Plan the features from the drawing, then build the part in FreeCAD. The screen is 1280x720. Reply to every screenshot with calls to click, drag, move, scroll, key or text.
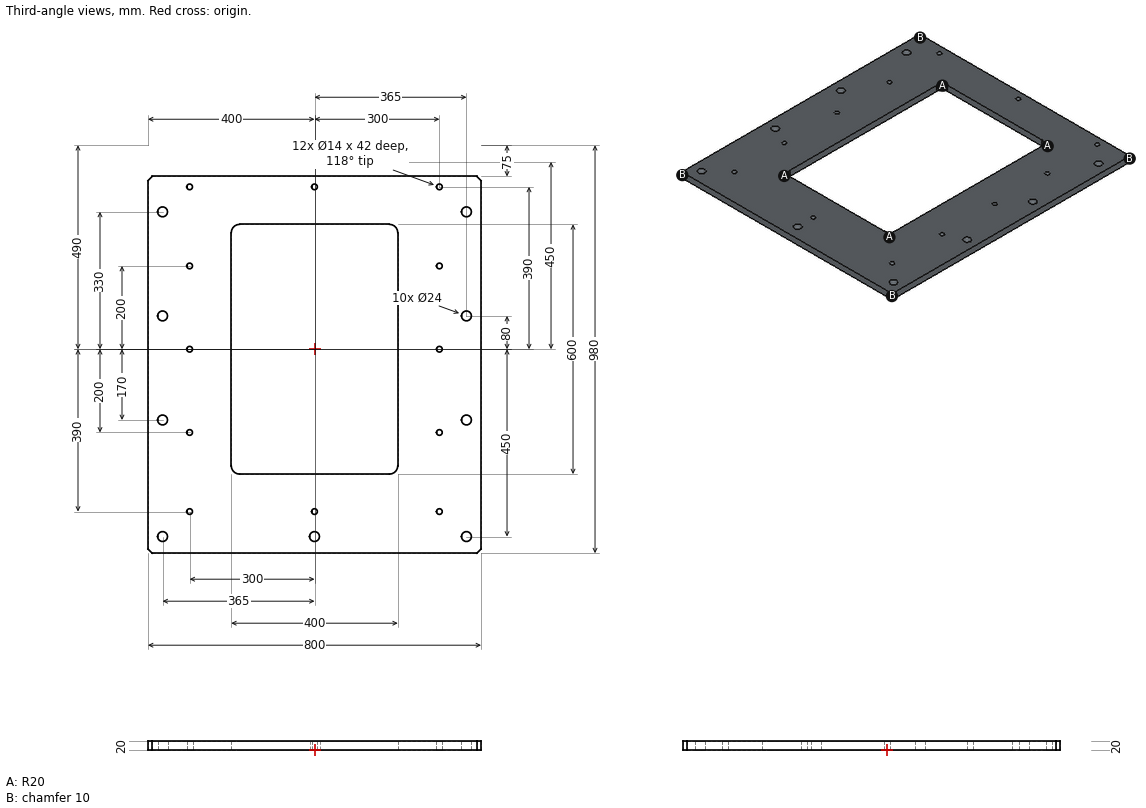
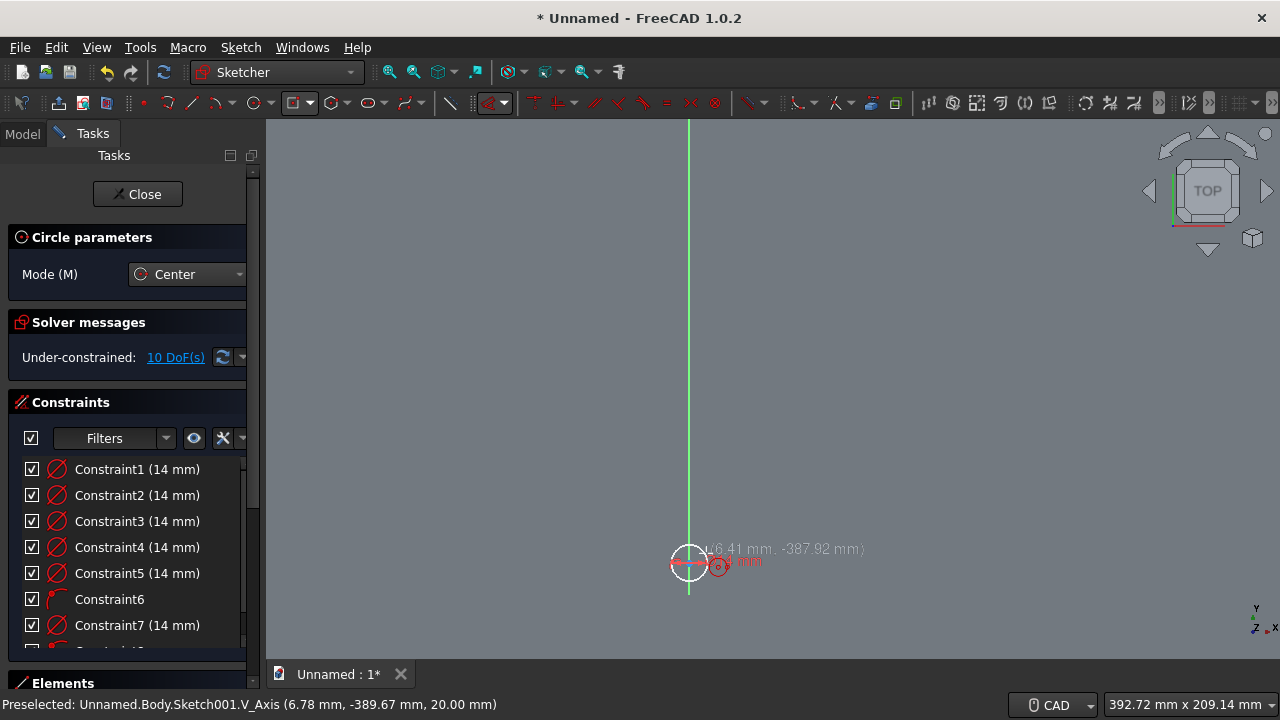
scroll(707, 555, down, 9)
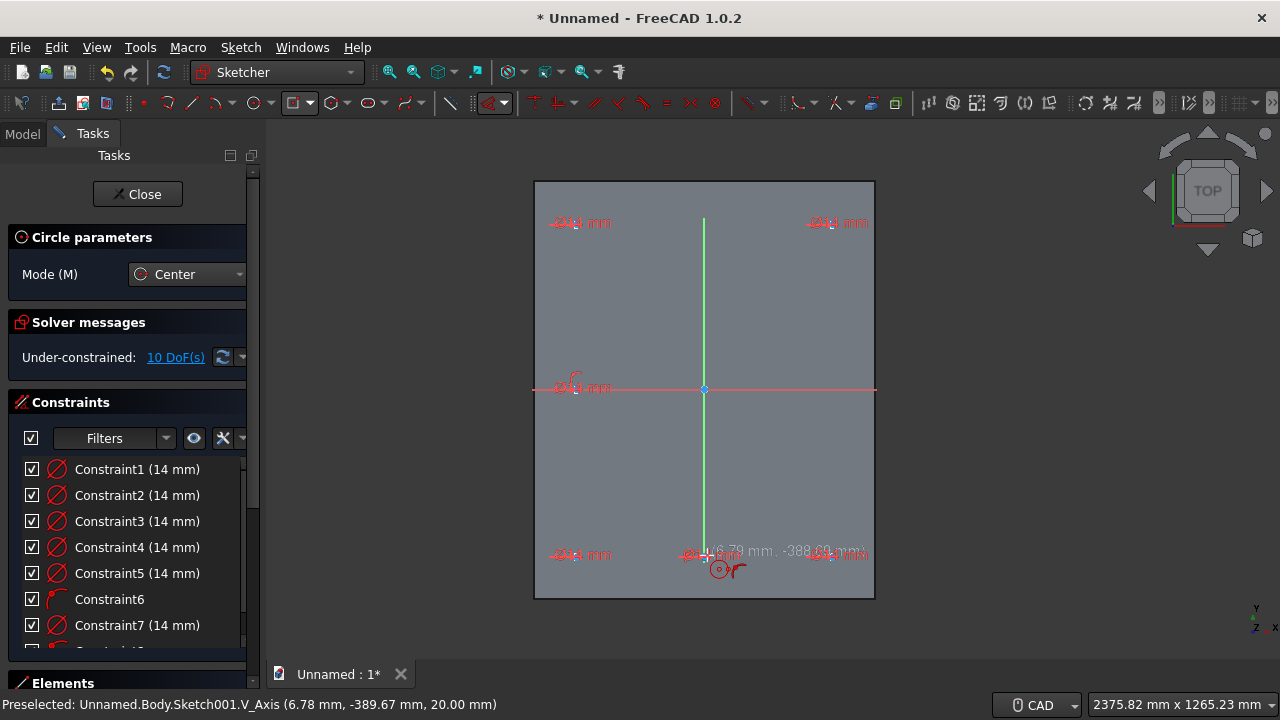
scroll(833, 390, up, 11)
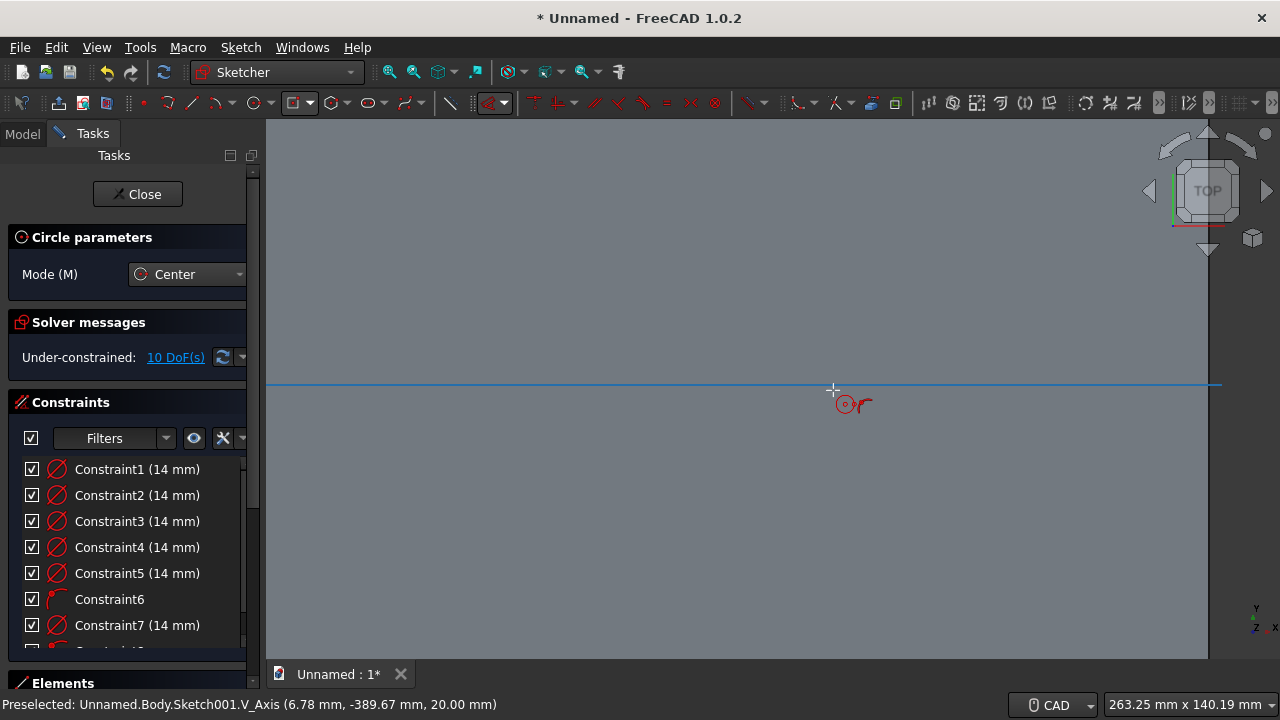
scroll(834, 389, down, 11)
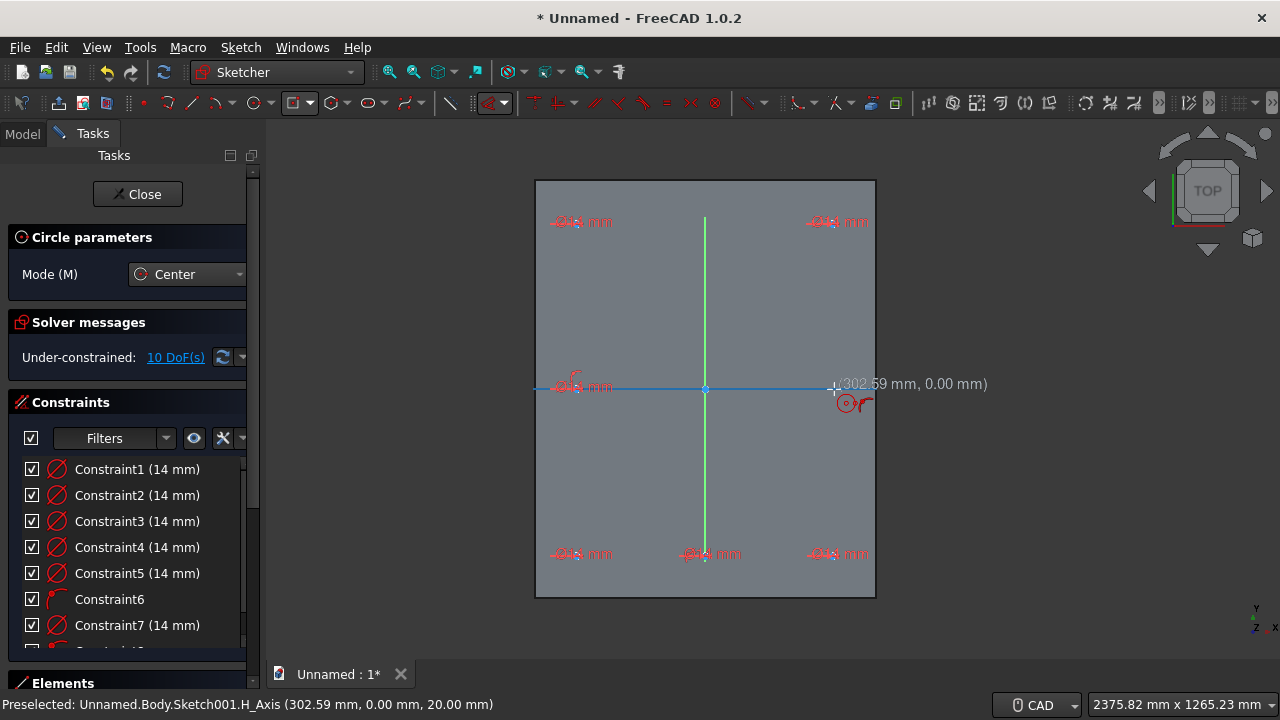
click(833, 389)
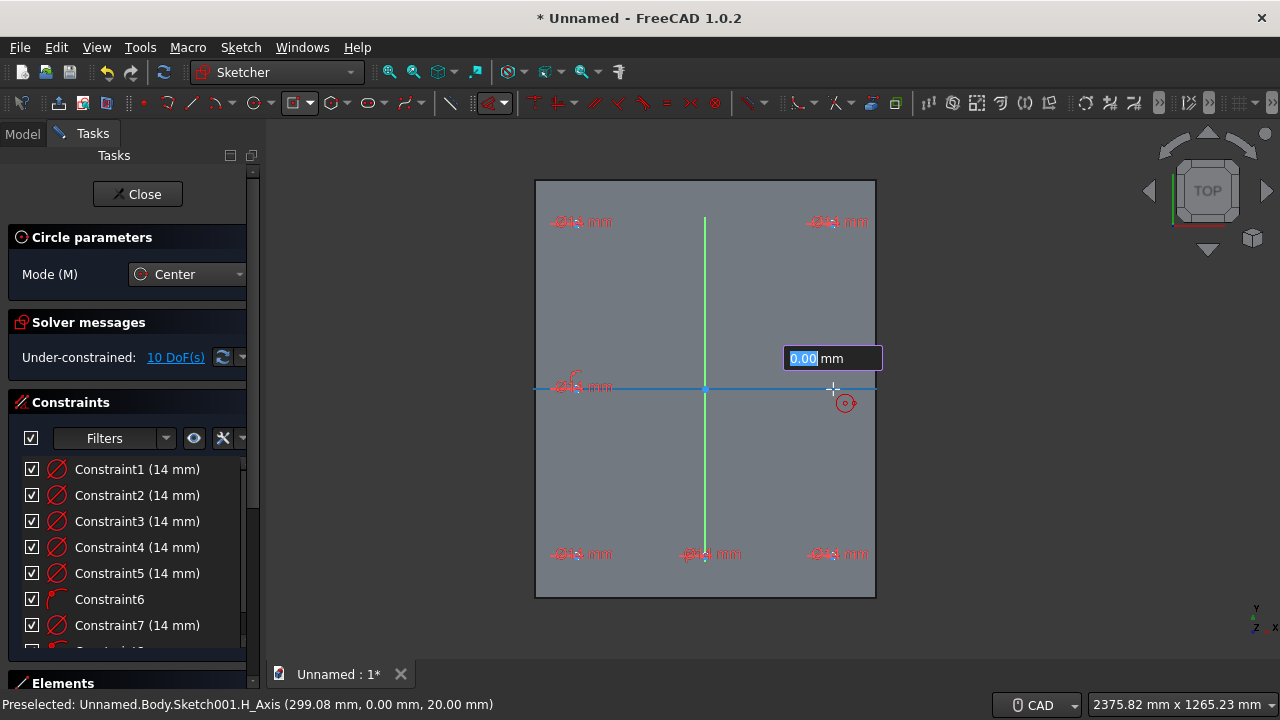
scroll(834, 386, up, 9)
move(834, 385)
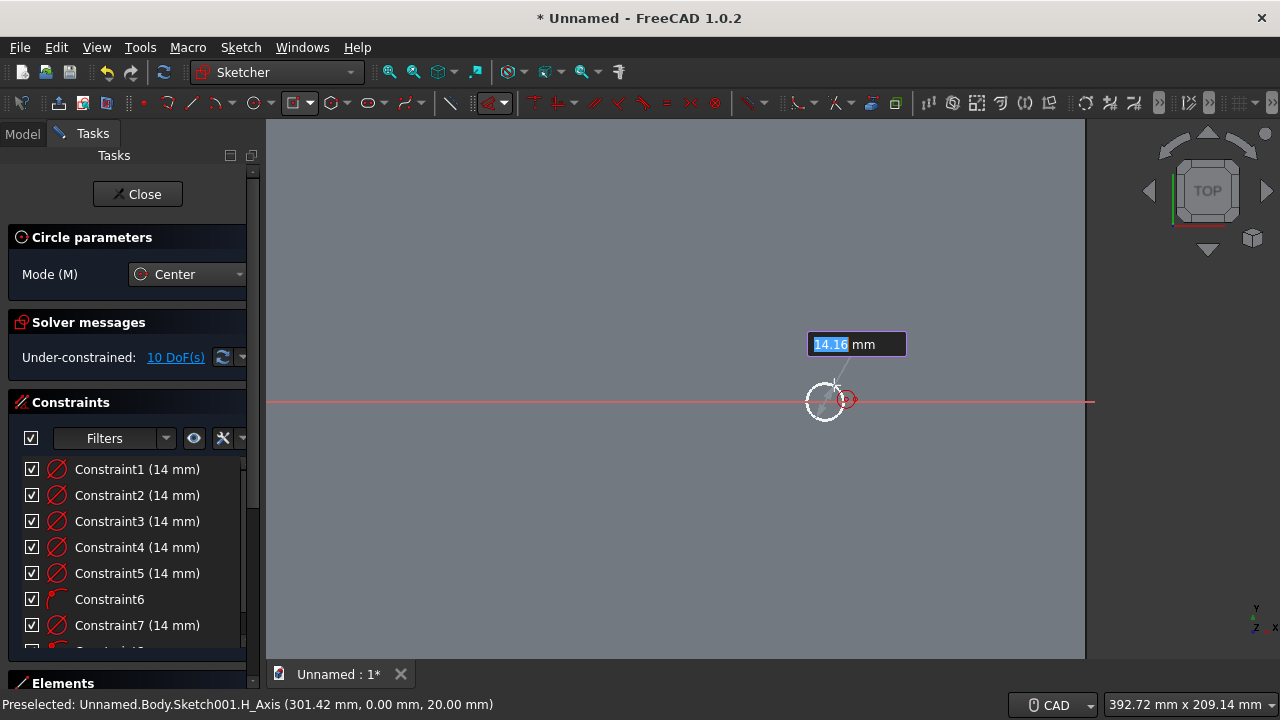
text(14)
key(Return)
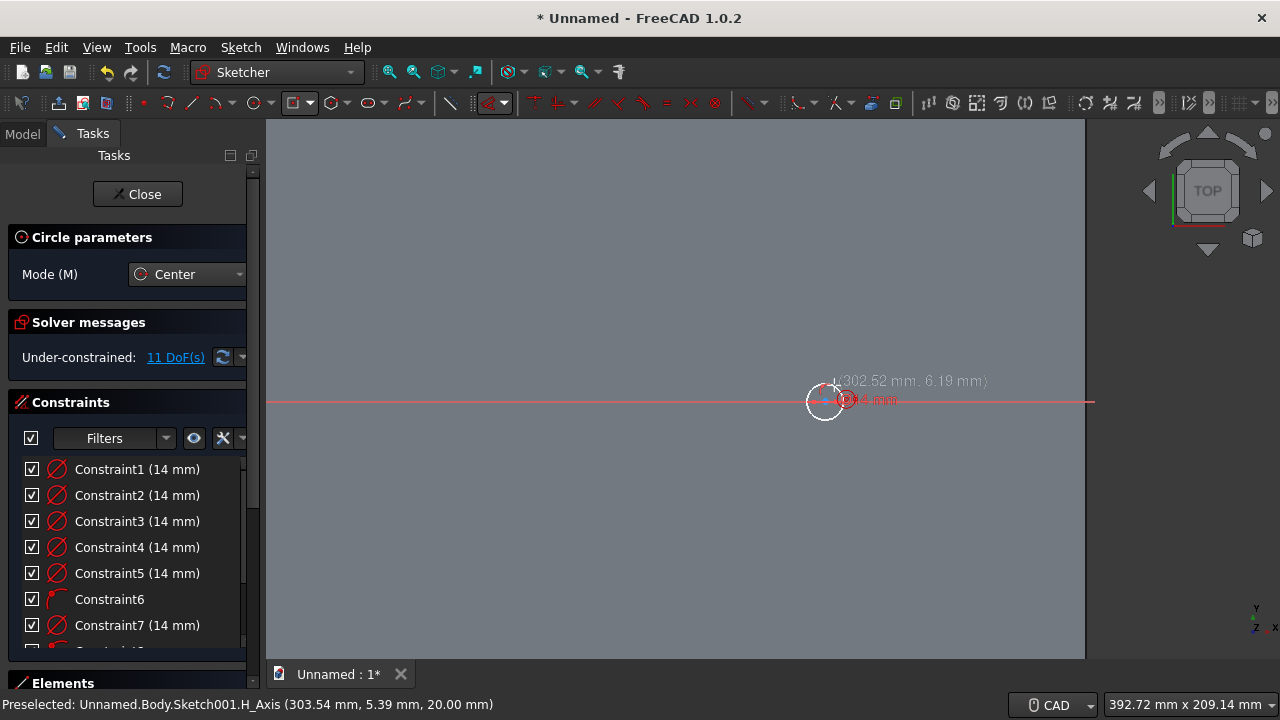
scroll(834, 386, down, 9)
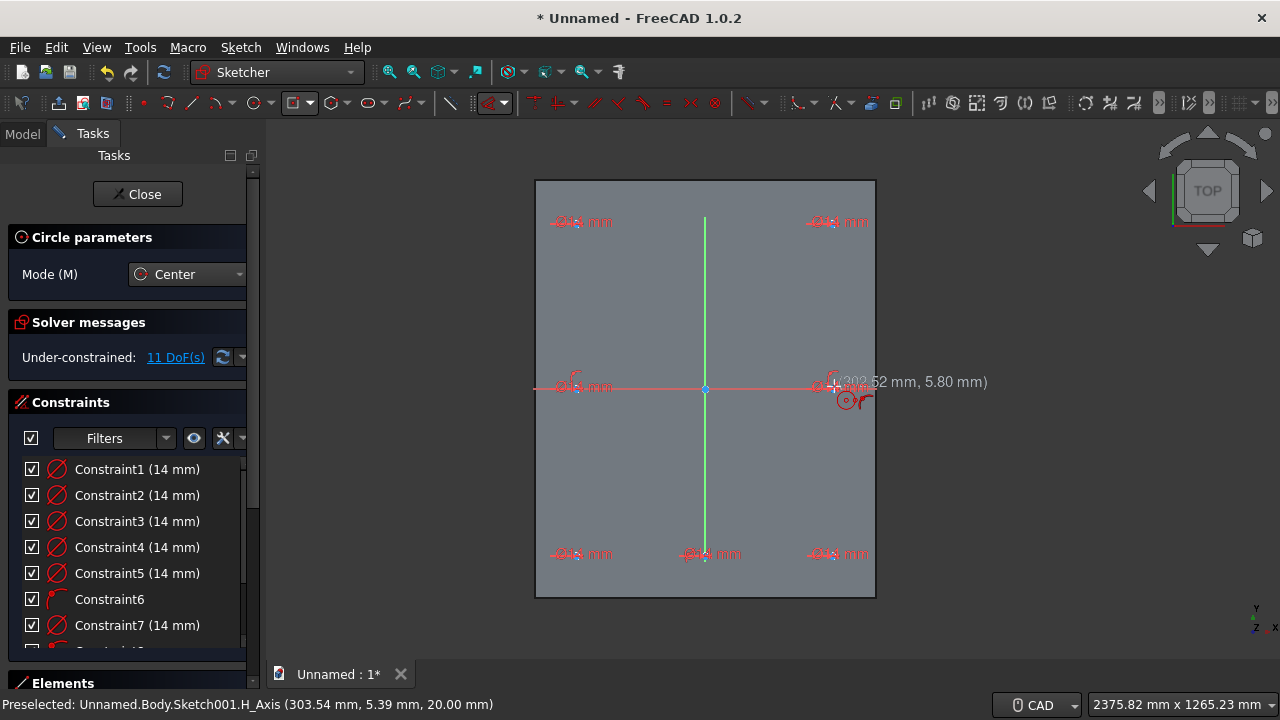
scroll(705, 223, up, 11)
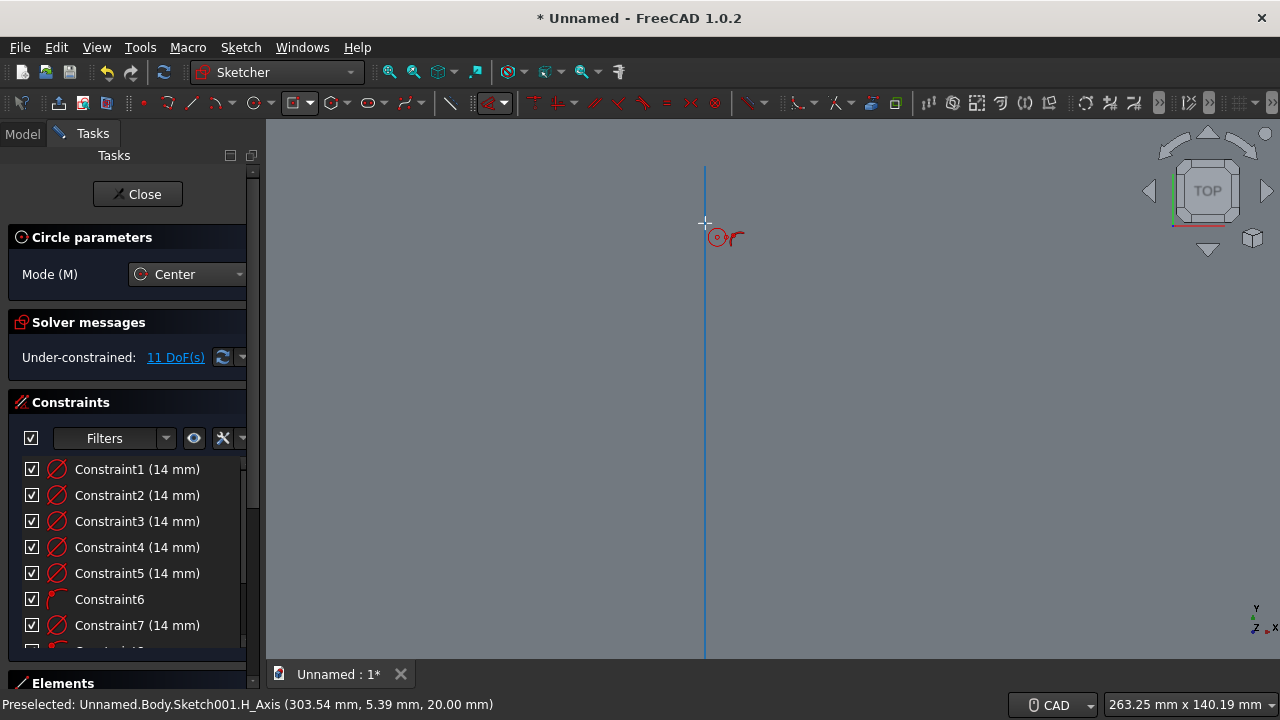
scroll(704, 223, down, 11)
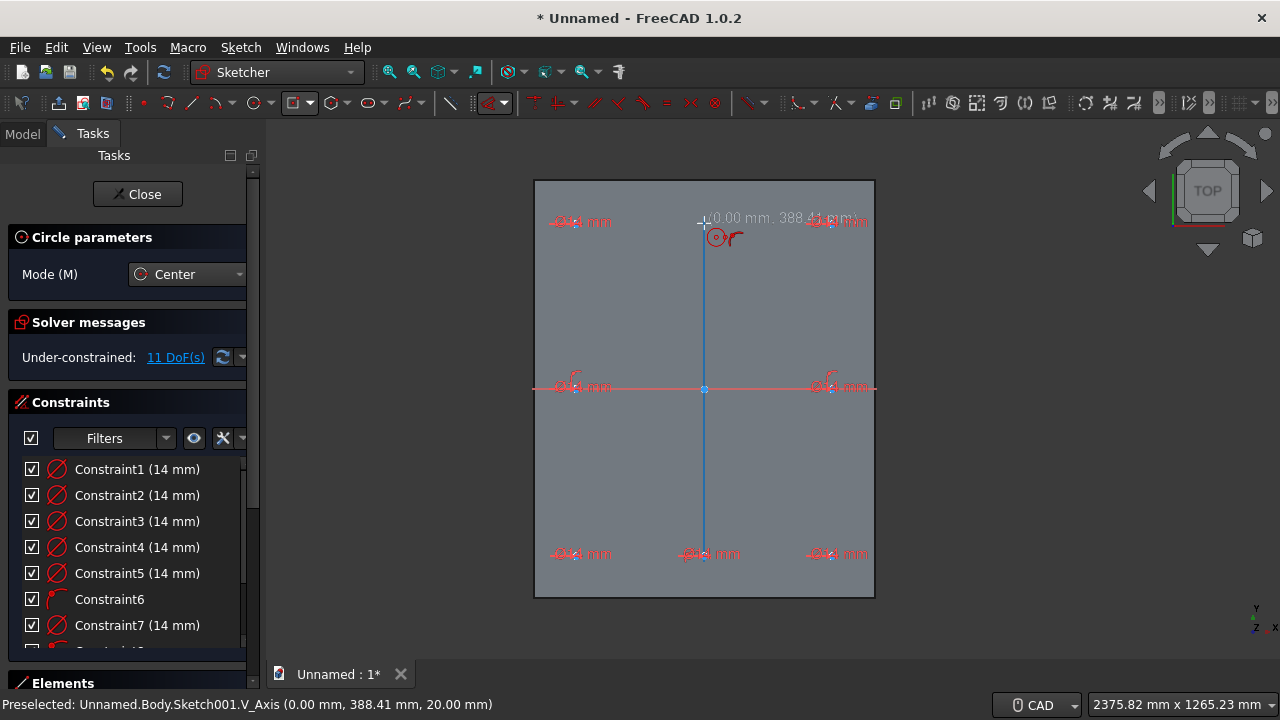
click(704, 223)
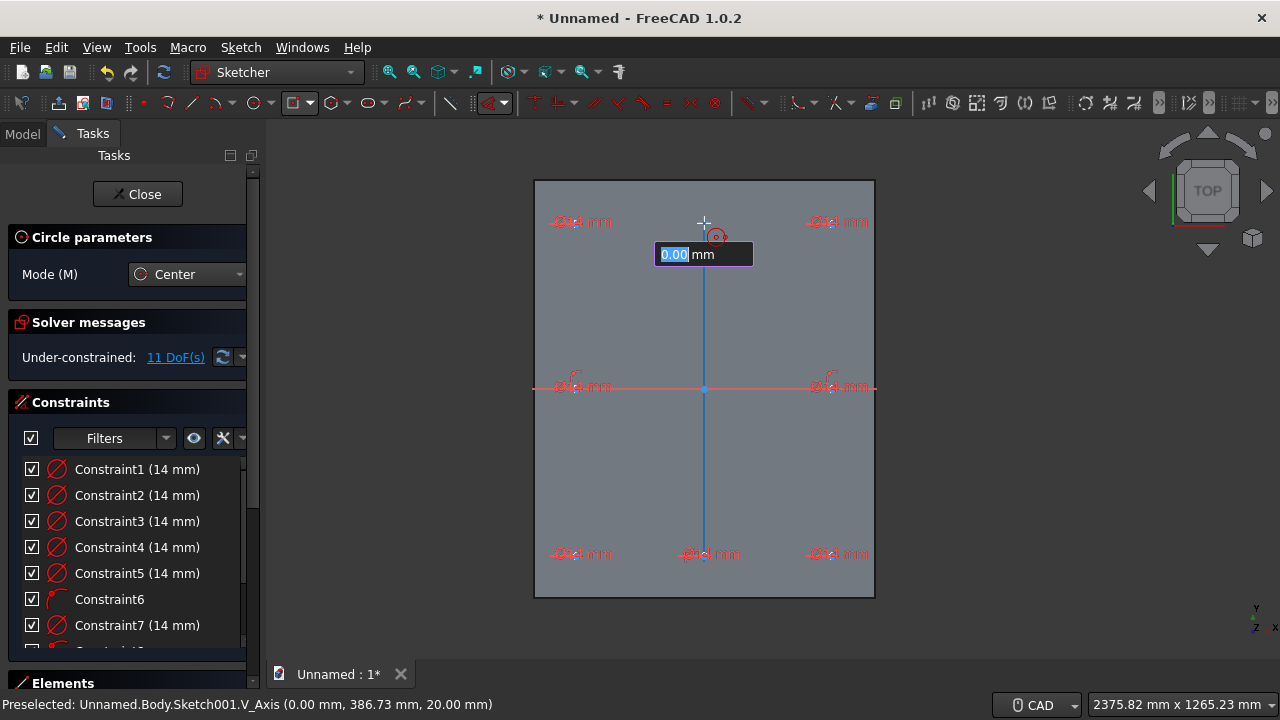
scroll(707, 222, up, 9)
move(706, 218)